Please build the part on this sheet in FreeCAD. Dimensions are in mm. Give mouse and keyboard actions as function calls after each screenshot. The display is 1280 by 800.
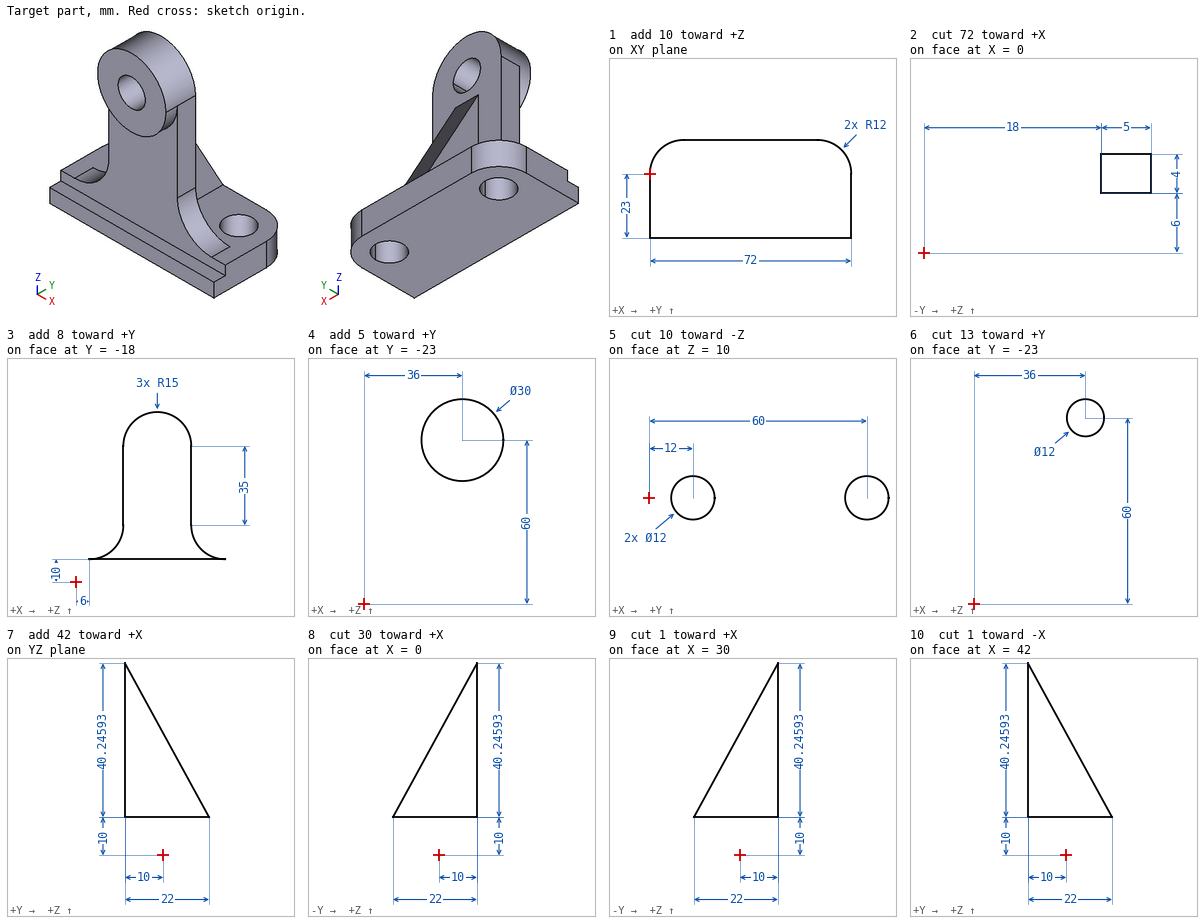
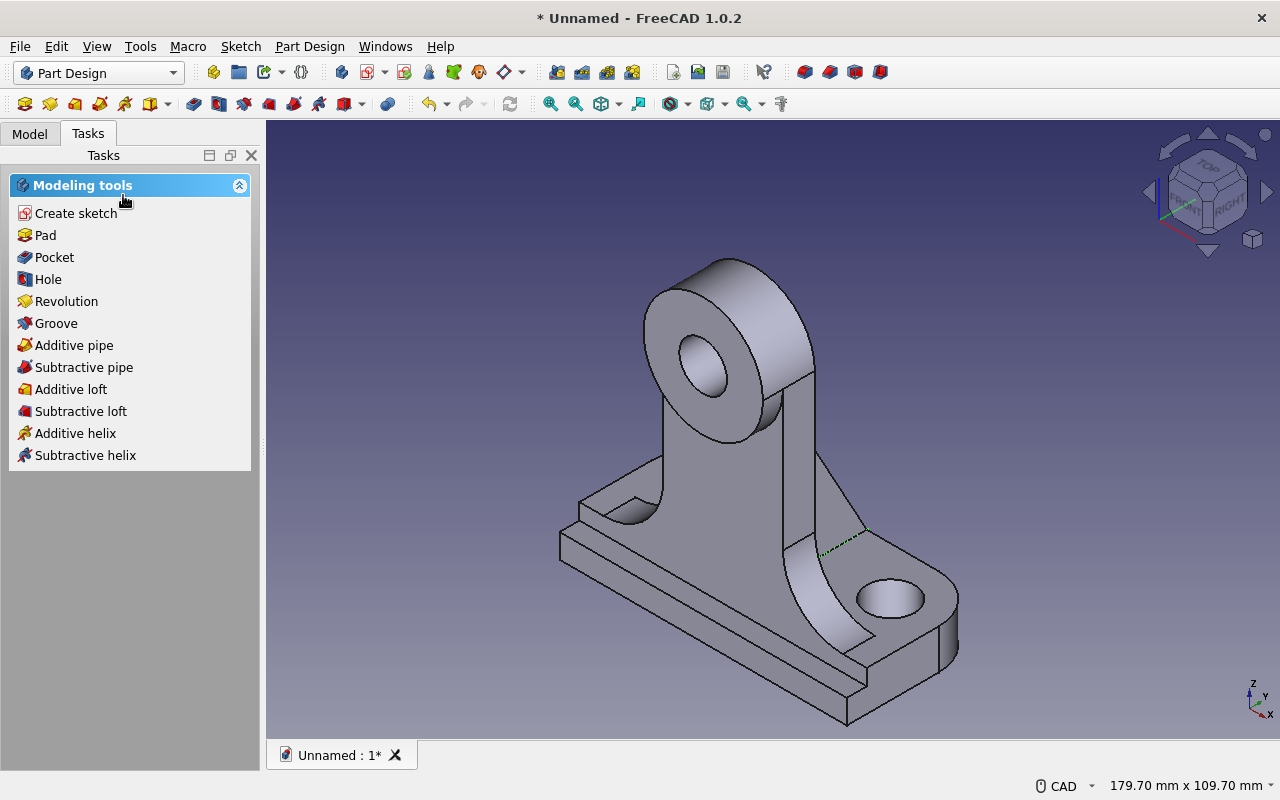
click(194, 104)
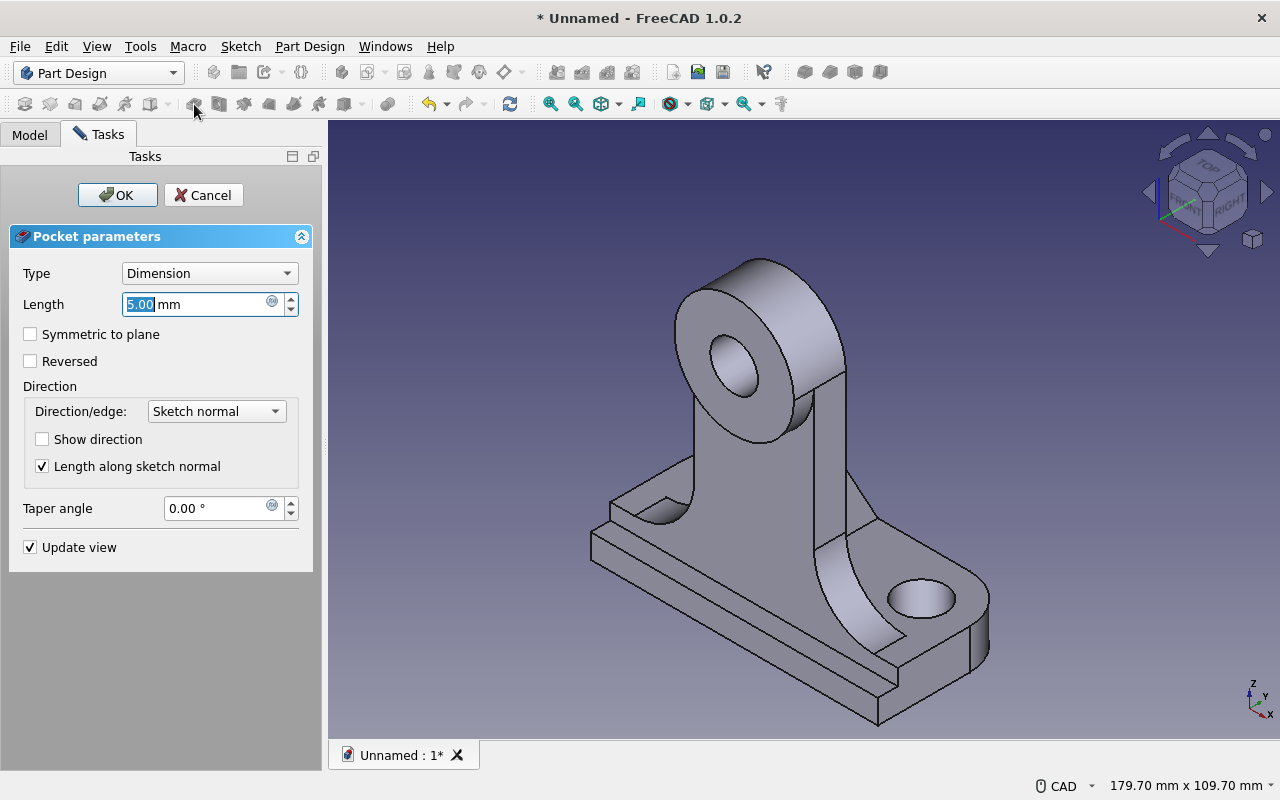
text(1)
key(Tab)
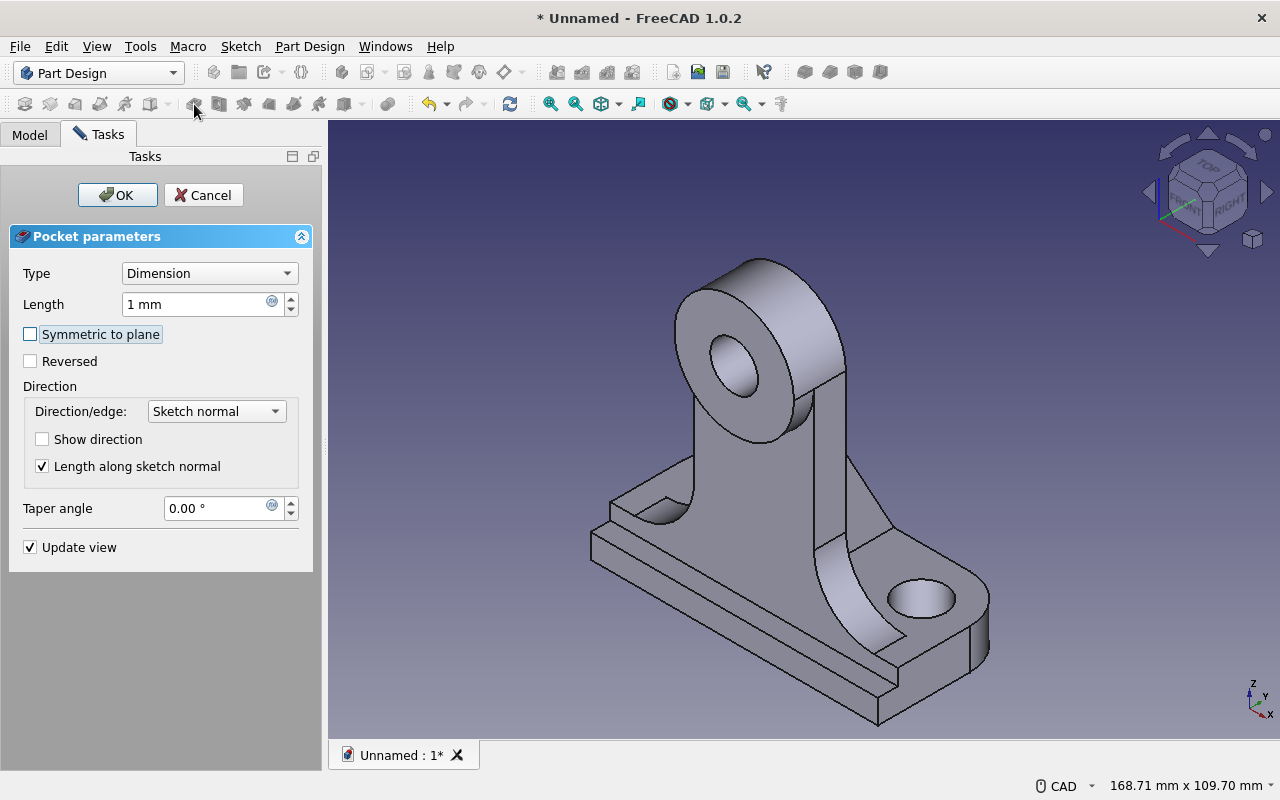
click(118, 195)